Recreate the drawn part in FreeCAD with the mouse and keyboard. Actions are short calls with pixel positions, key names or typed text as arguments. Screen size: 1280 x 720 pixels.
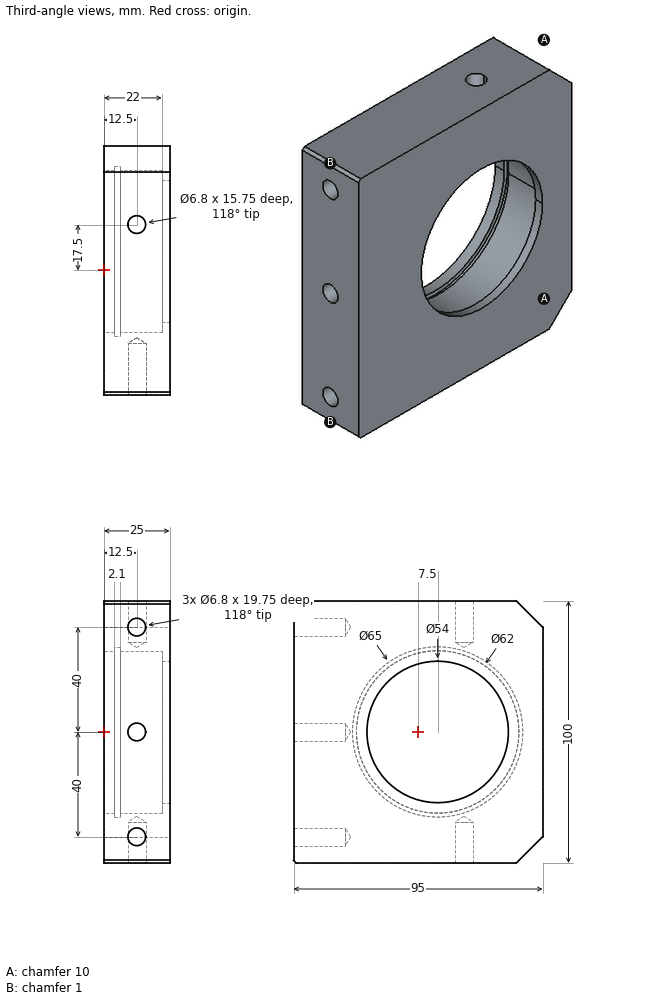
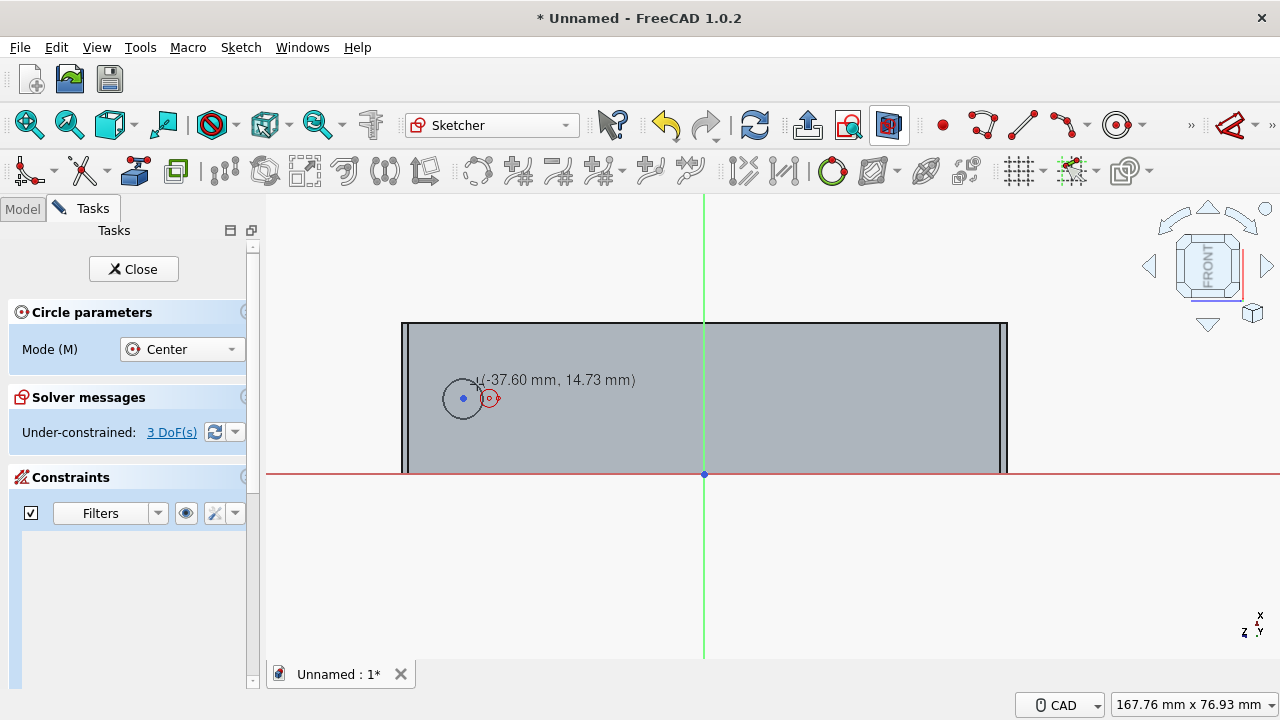
click(704, 398)
click(719, 384)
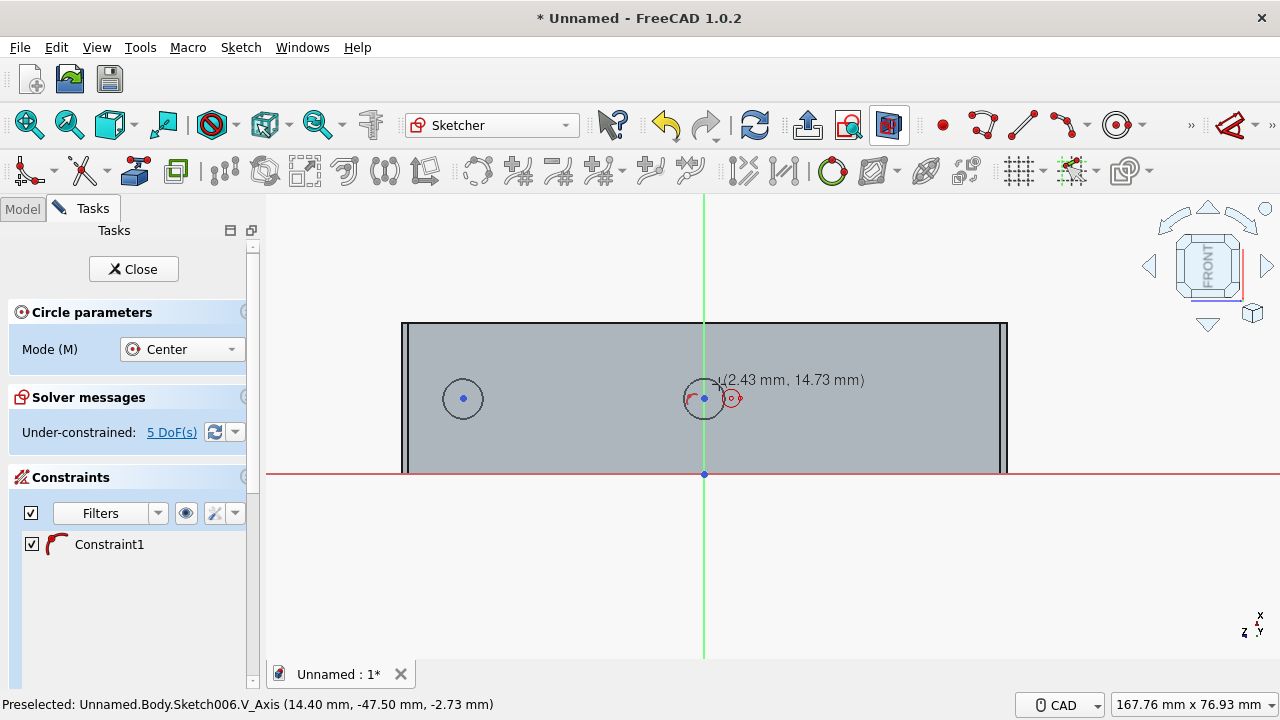
click(946, 398)
click(961, 384)
key(Escape)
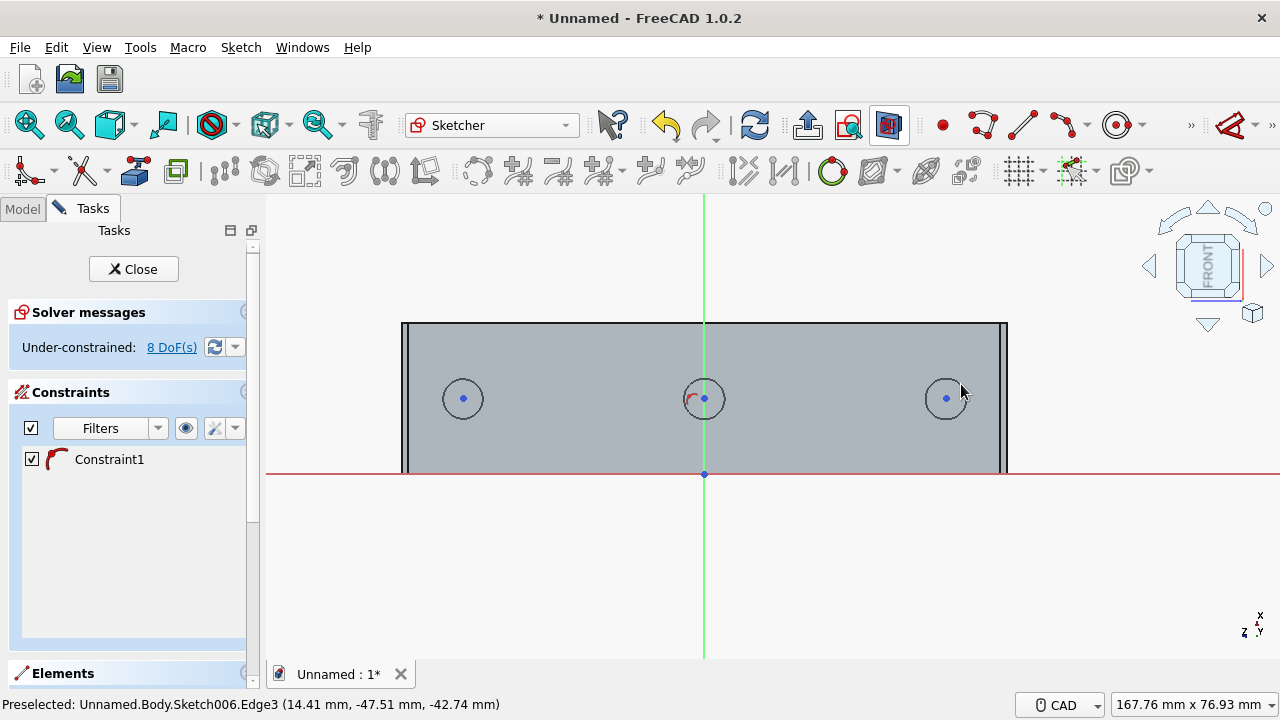
click(477, 385)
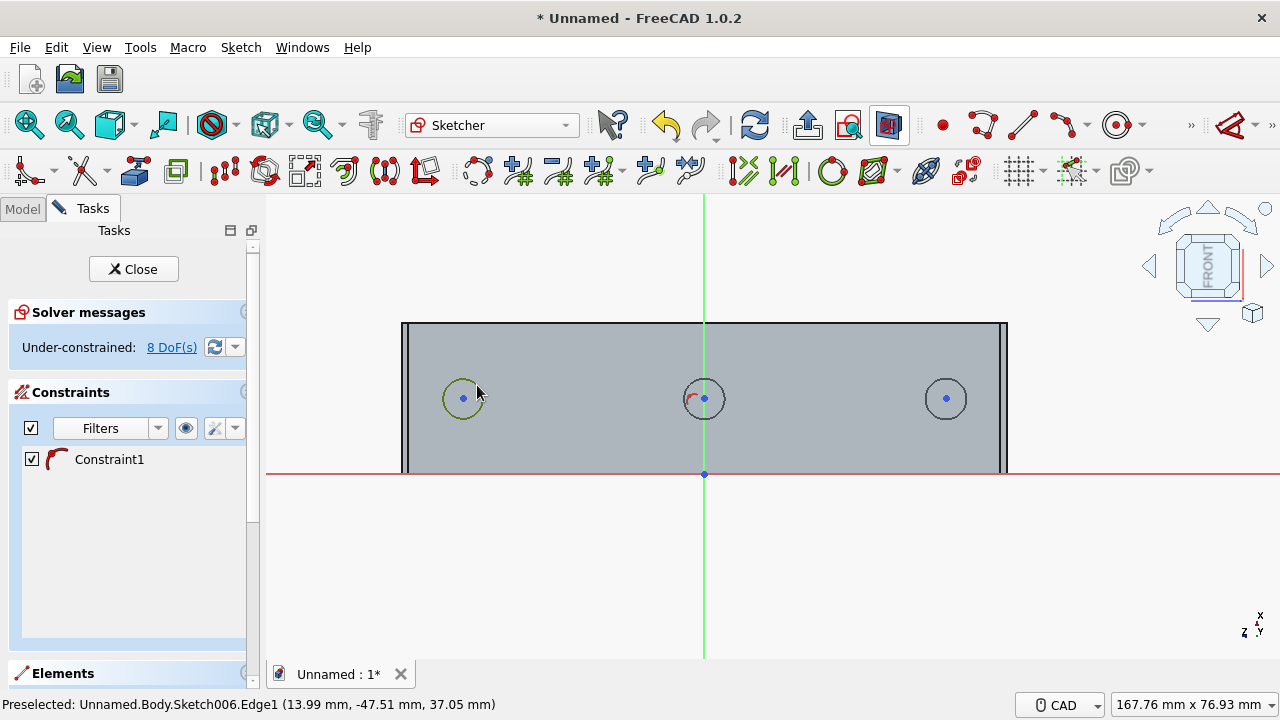
click(719, 385)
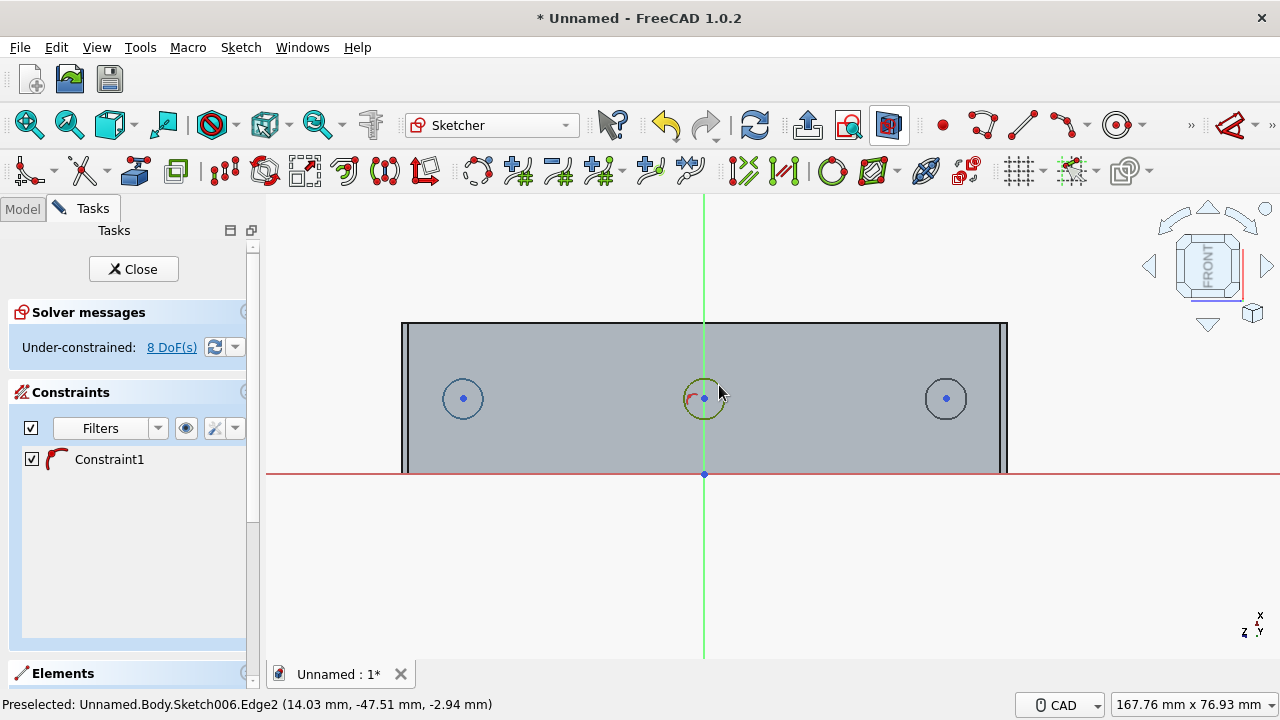
click(960, 384)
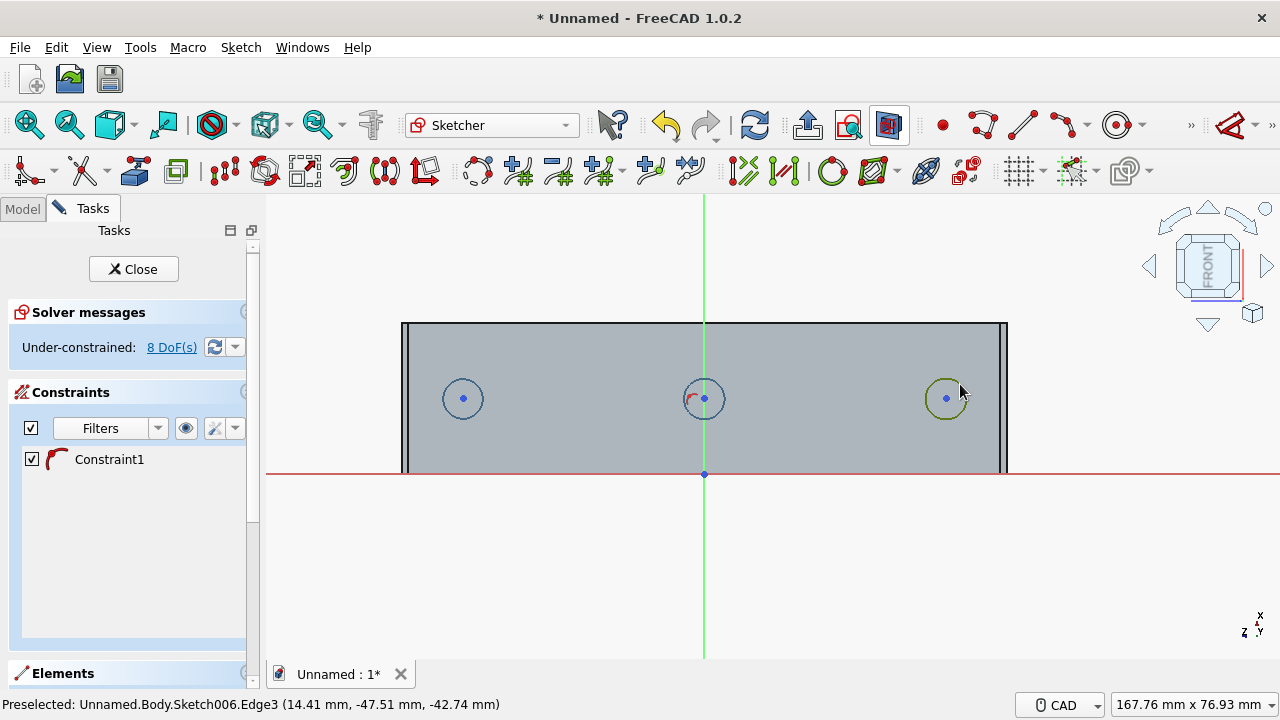
key(e)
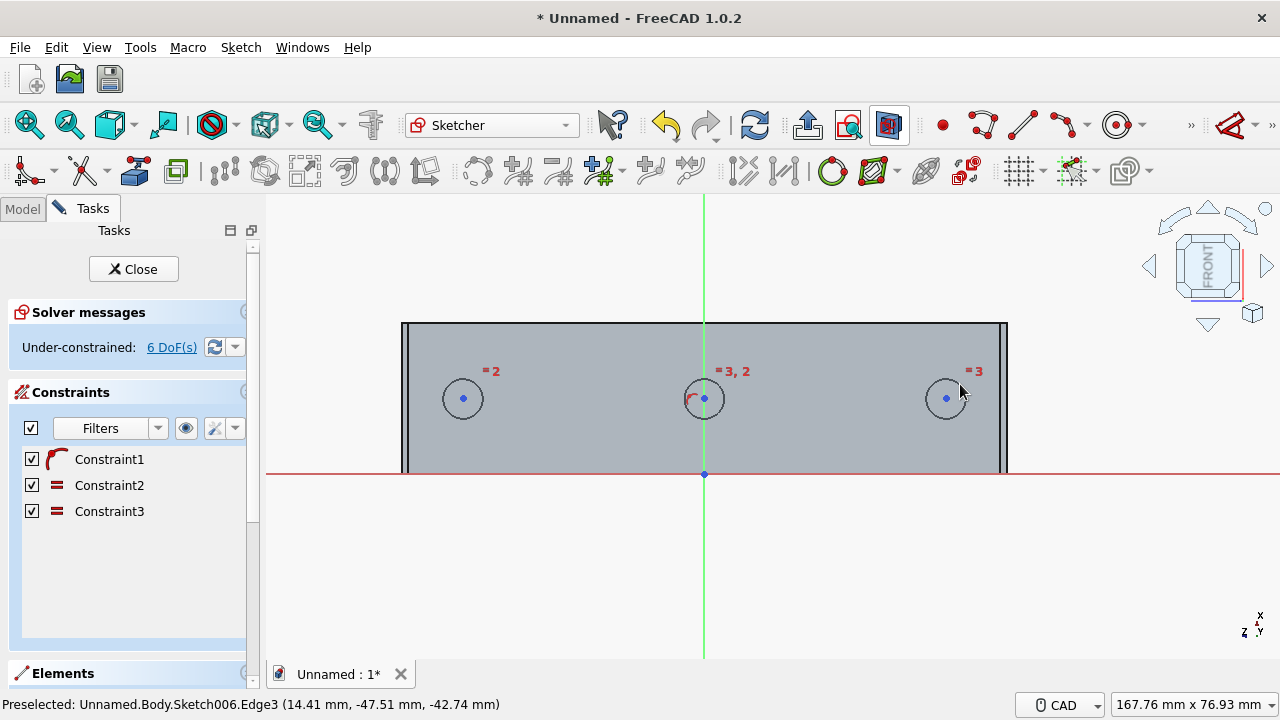
click(1230, 126)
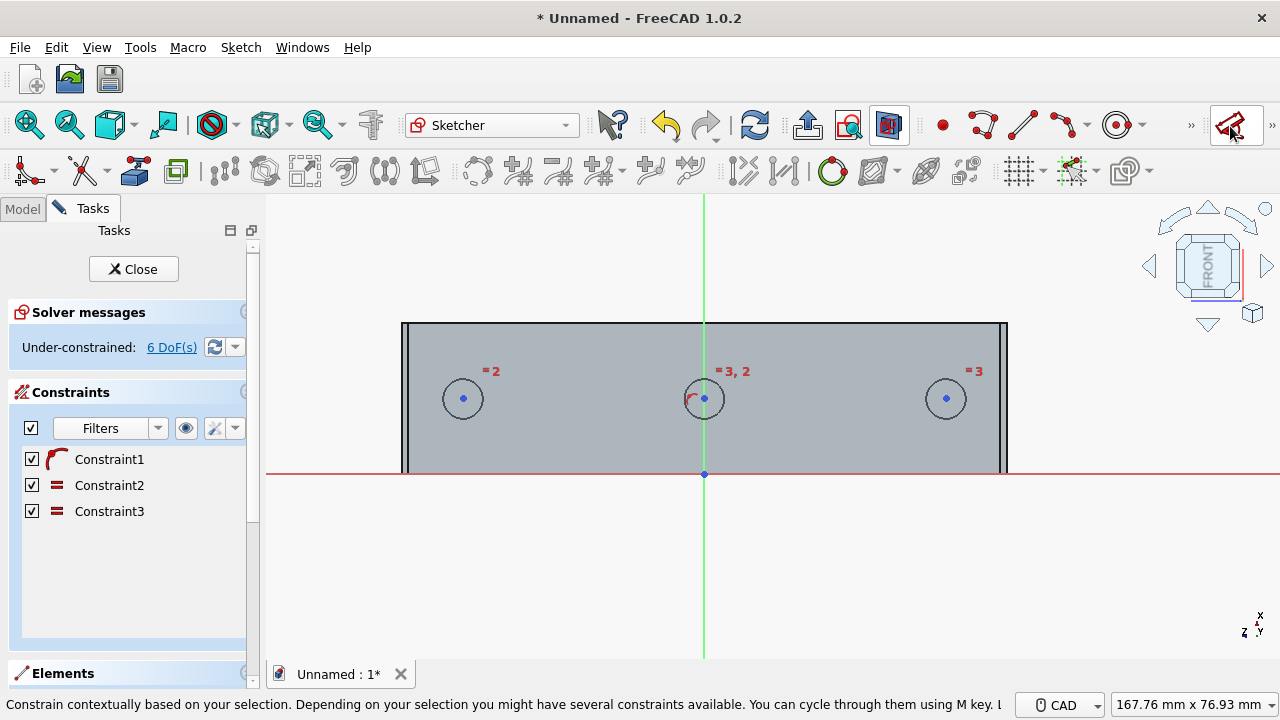
click(477, 385)
click(500, 362)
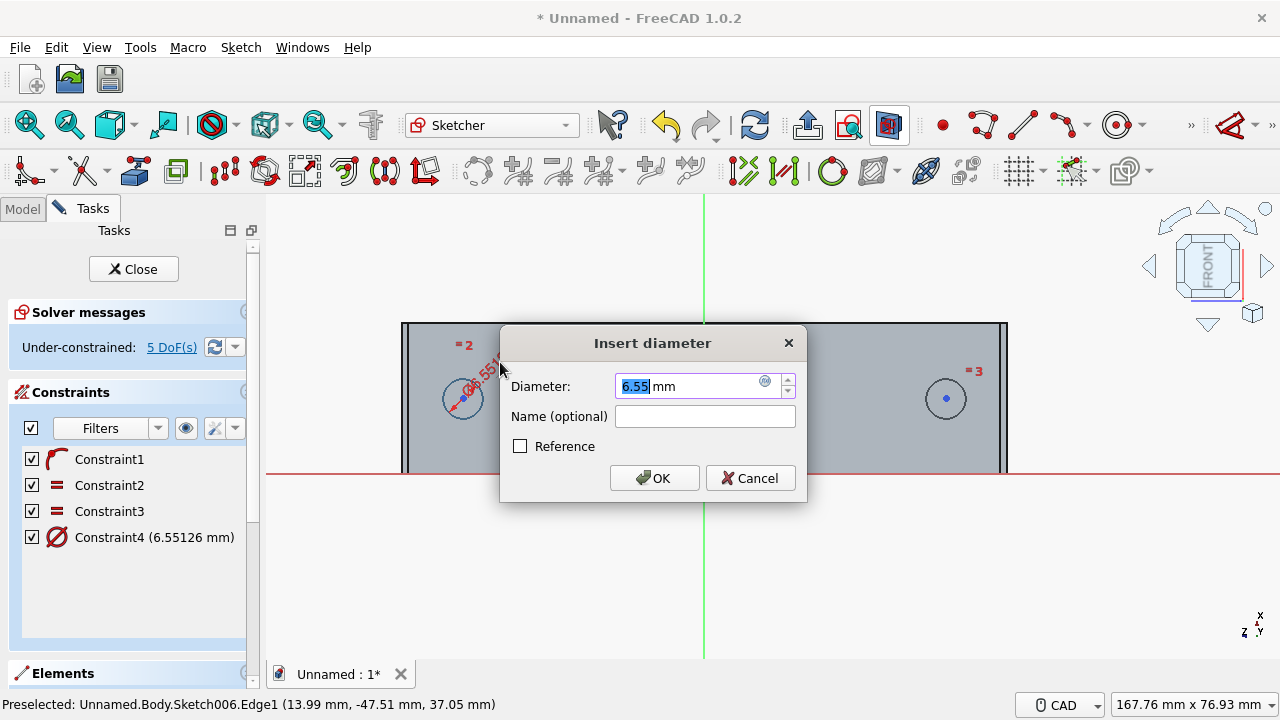
text(6.8)
key(Return)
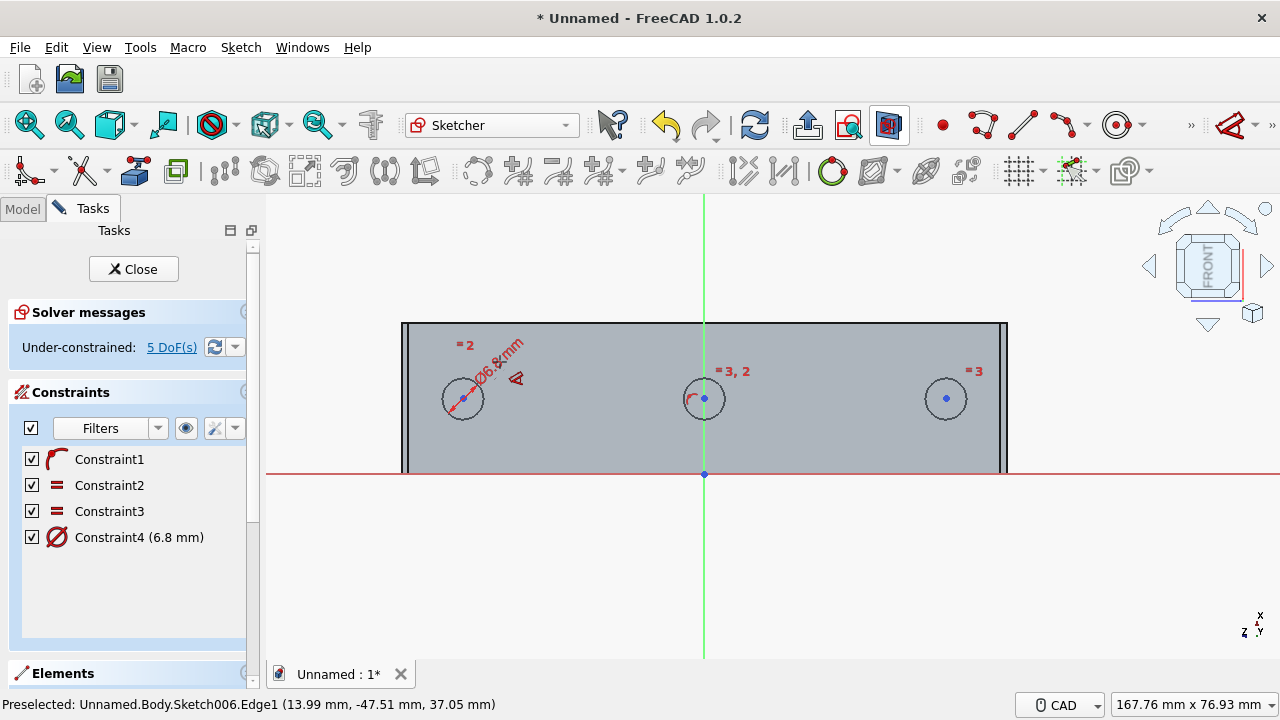
click(463, 399)
click(584, 508)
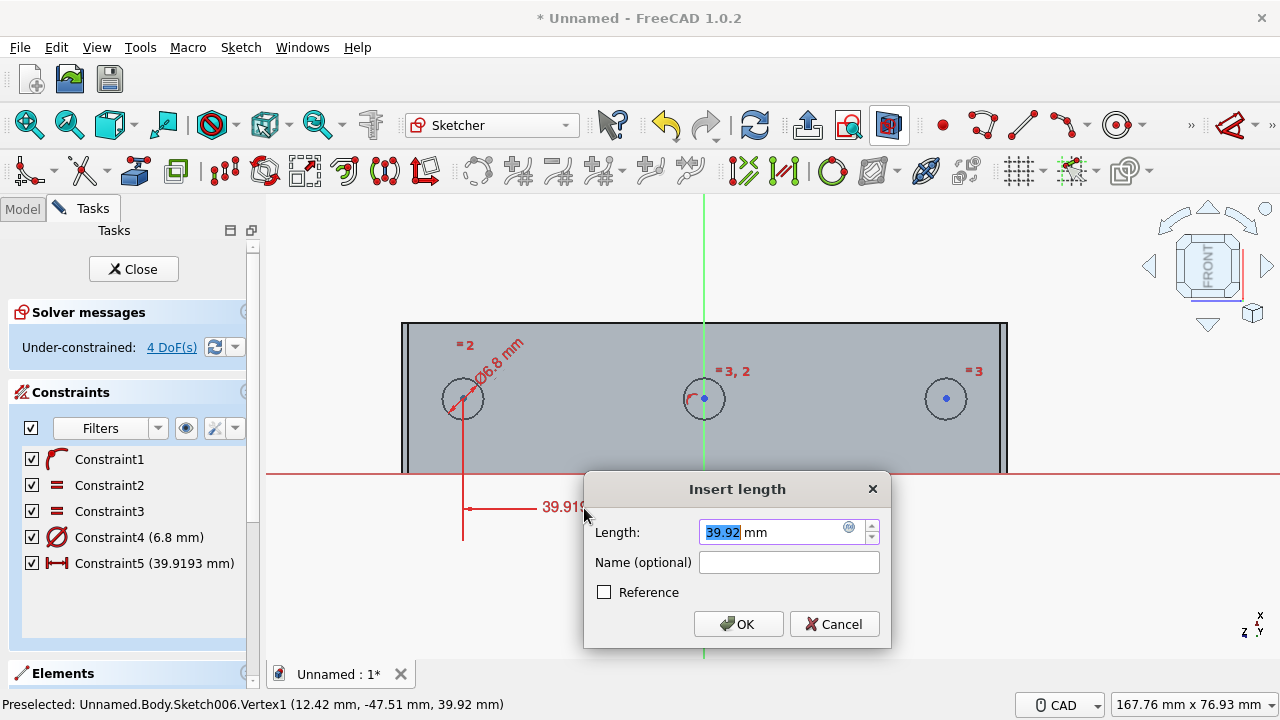
text(40)
key(Return)